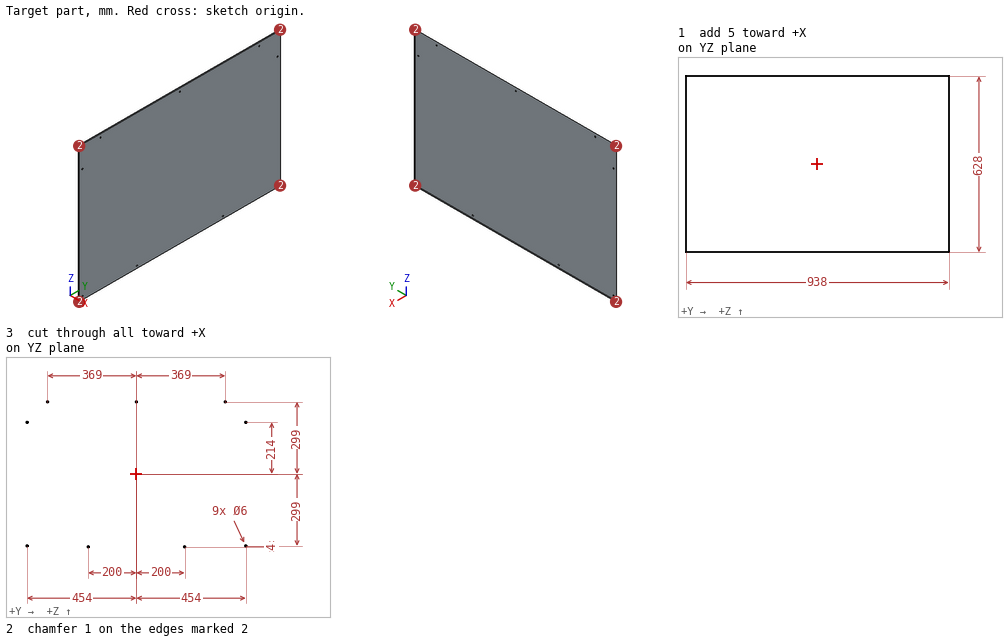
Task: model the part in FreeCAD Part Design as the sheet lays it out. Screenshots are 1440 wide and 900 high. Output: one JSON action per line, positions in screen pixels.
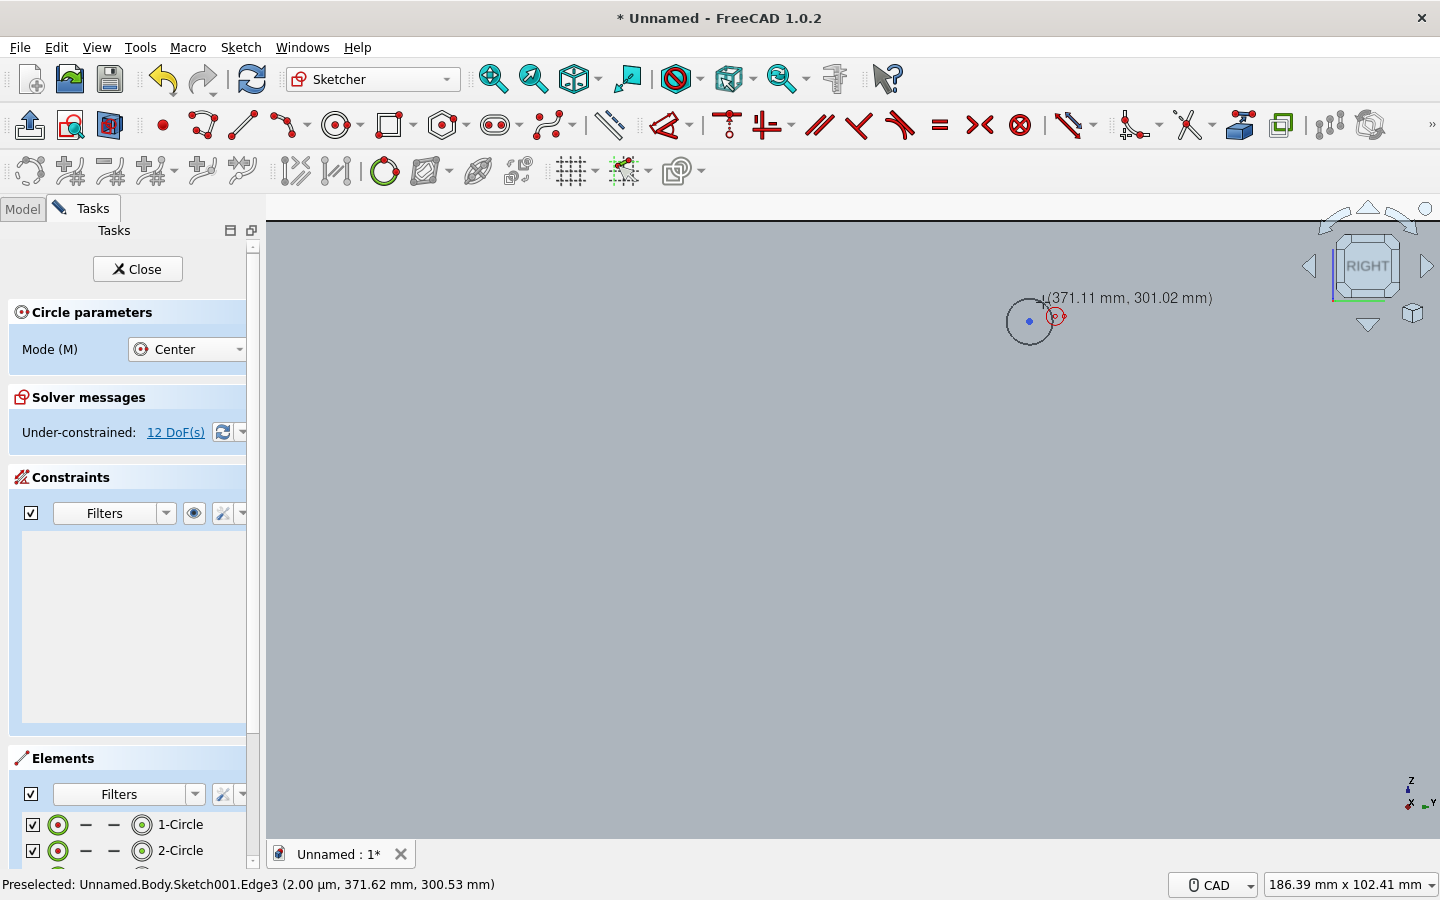
{"action": "scroll", "coordinate": [1044, 305], "scroll_direction": "down", "scroll_amount": 11}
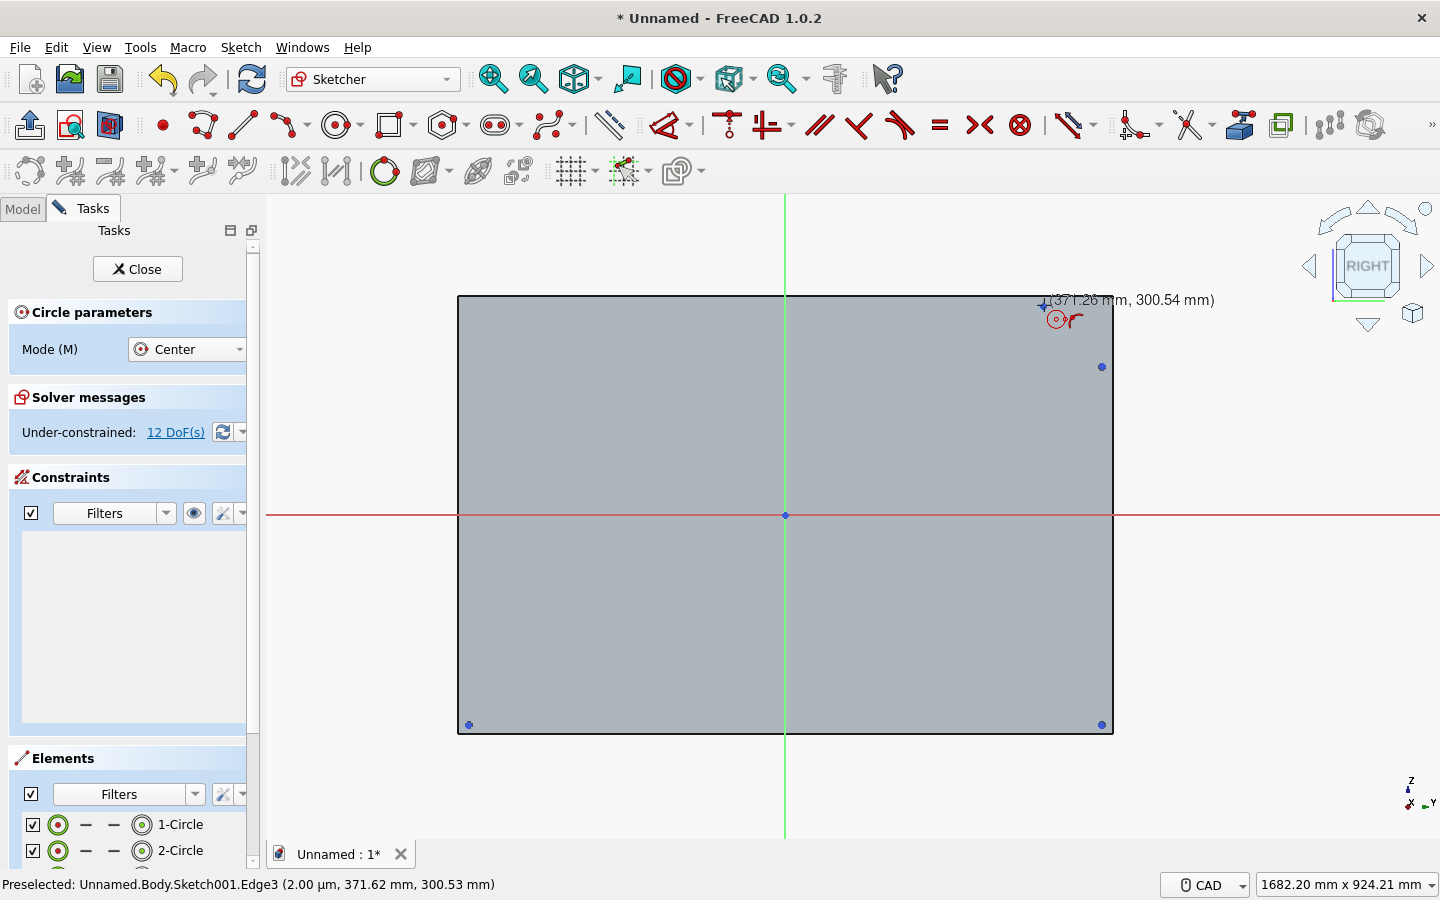
{"action": "scroll", "coordinate": [528, 306], "scroll_direction": "up", "scroll_amount": 12}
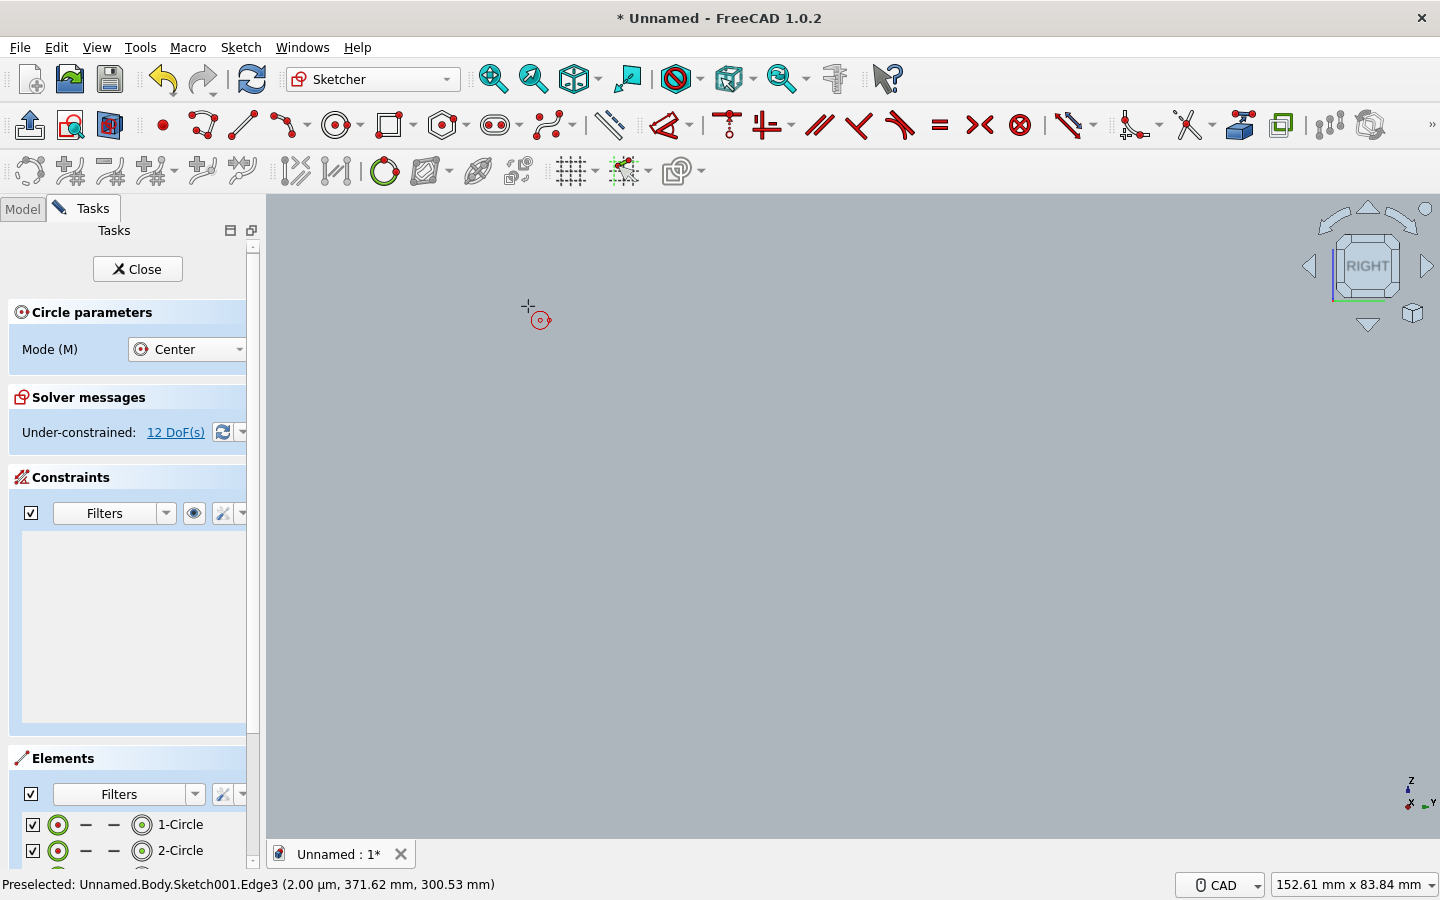
{"action": "scroll", "coordinate": [527, 306], "scroll_direction": "down", "scroll_amount": 12}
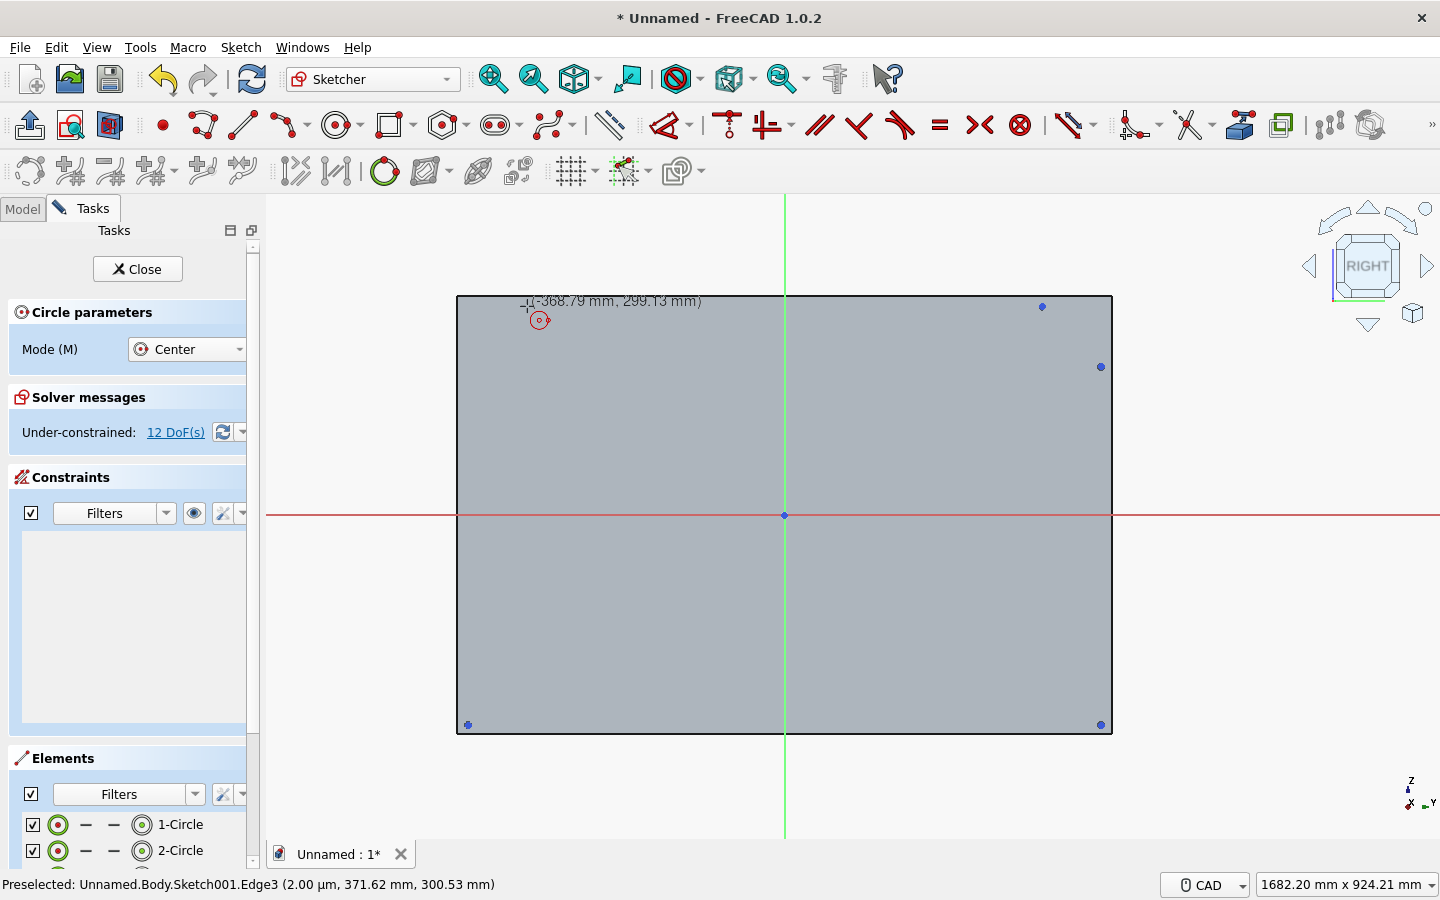
{"action": "left_click", "coordinate": [527, 306]}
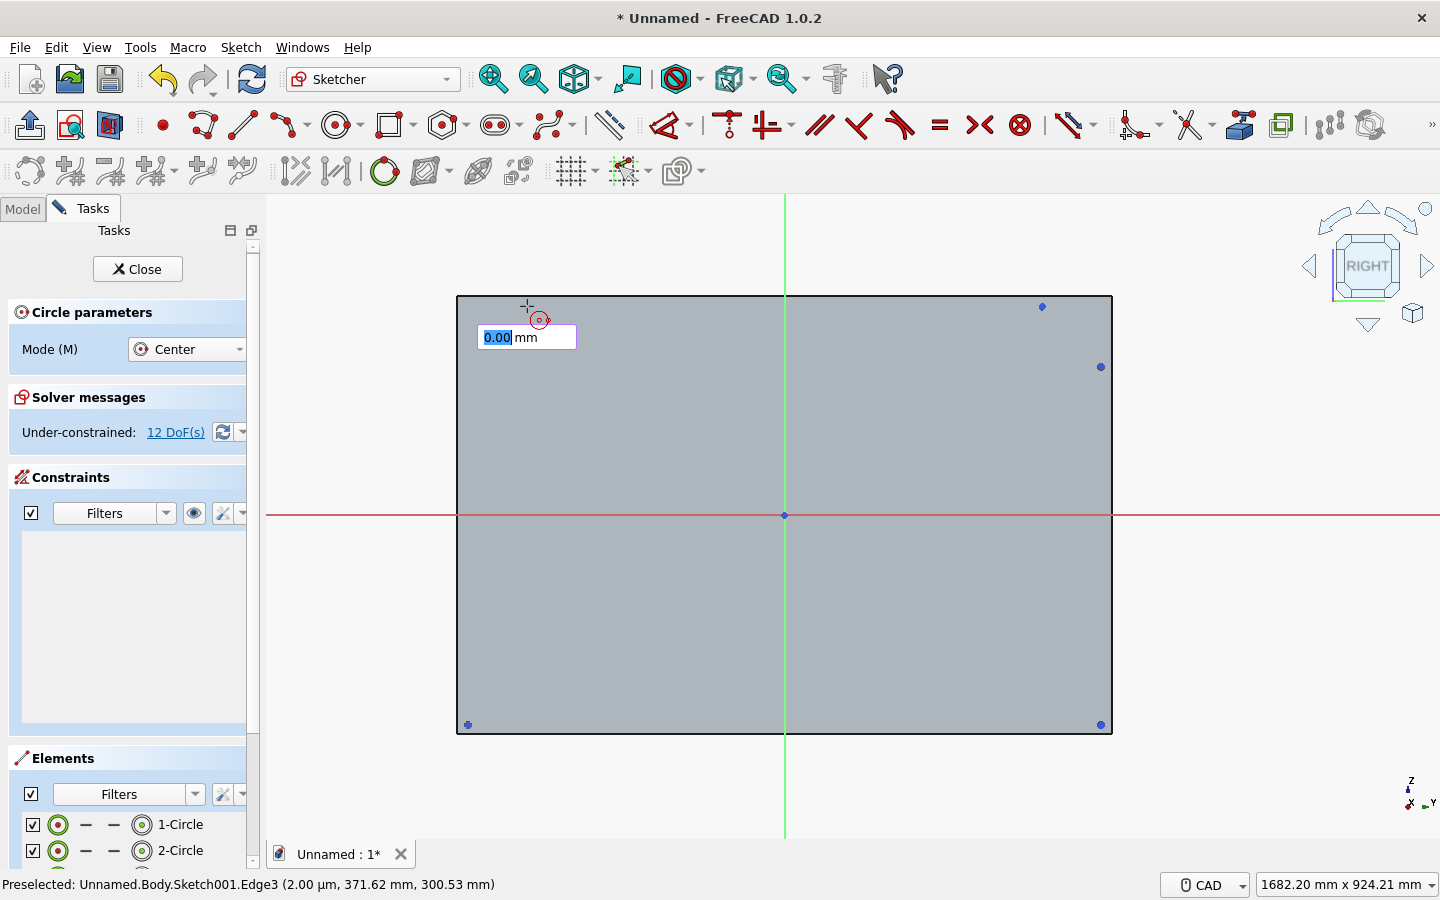
{"action": "scroll", "coordinate": [529, 305], "scroll_direction": "up", "scroll_amount": 11}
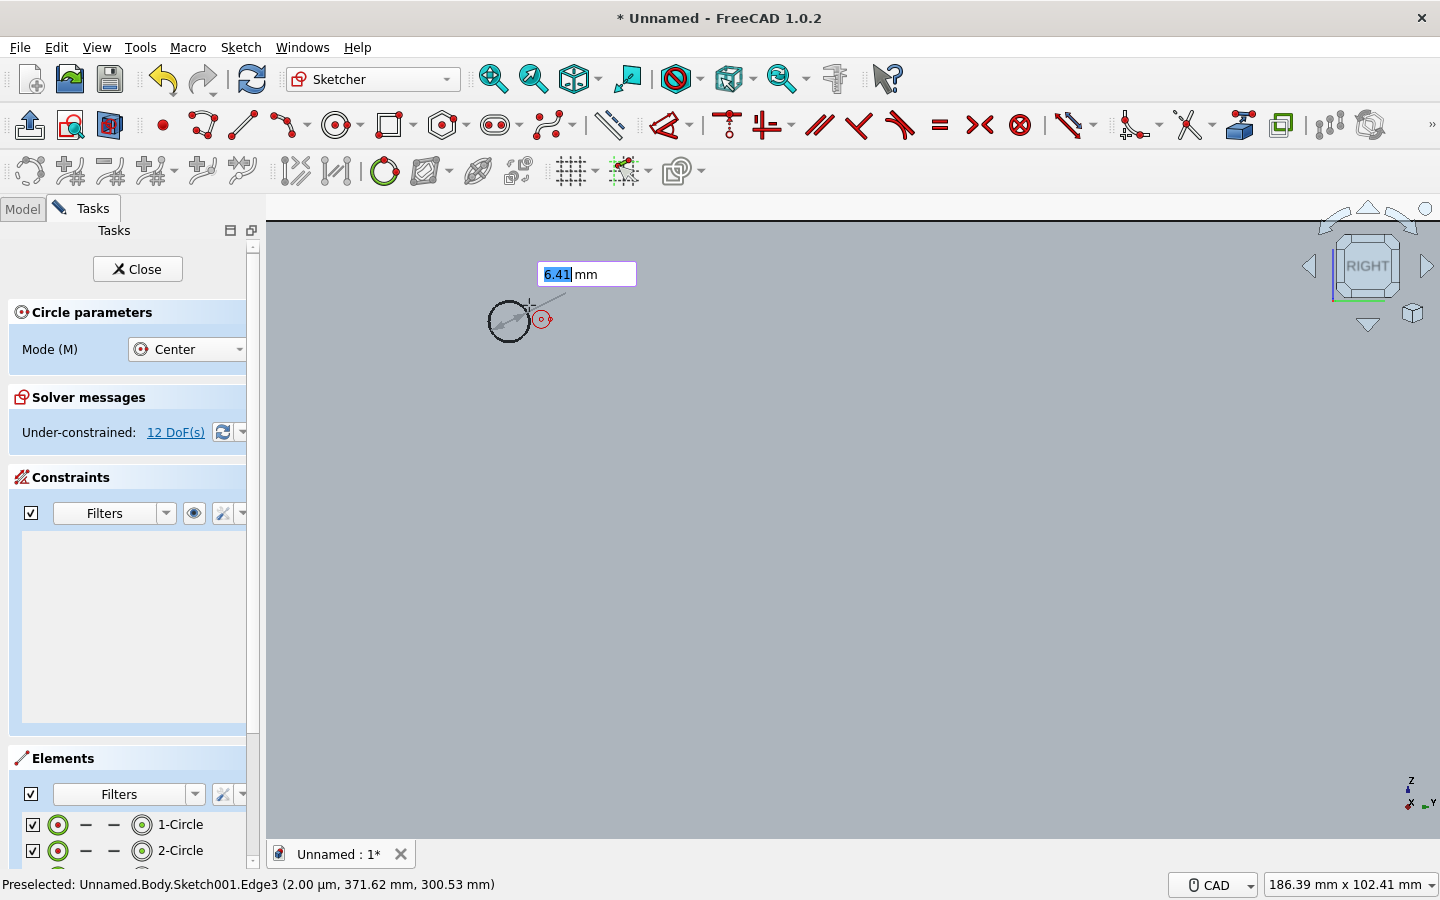
{"action": "left_click", "coordinate": [523, 302]}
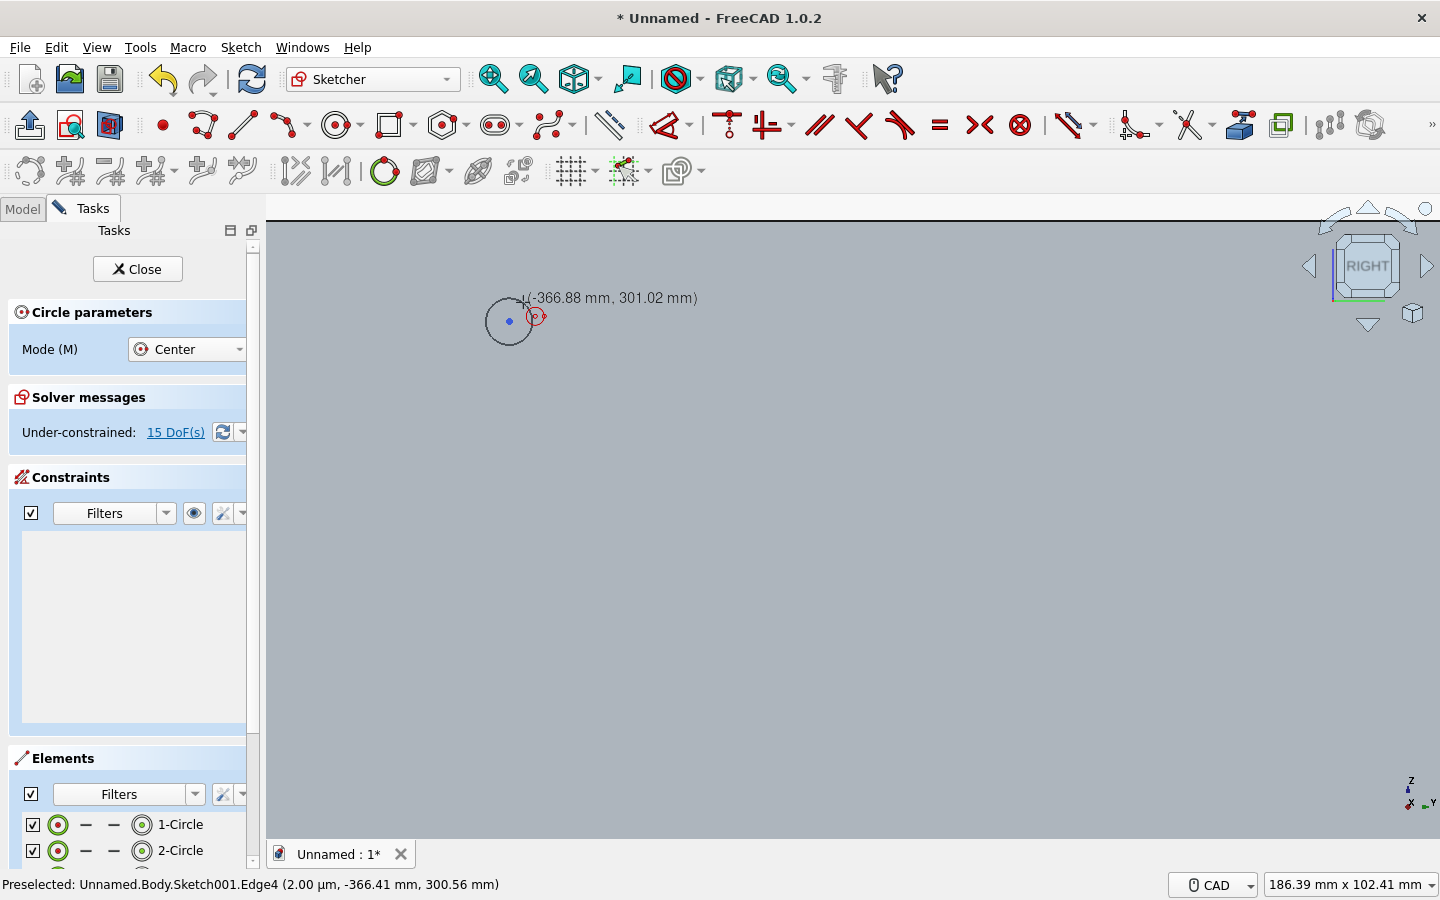
{"action": "scroll", "coordinate": [529, 305], "scroll_direction": "down", "scroll_amount": 11}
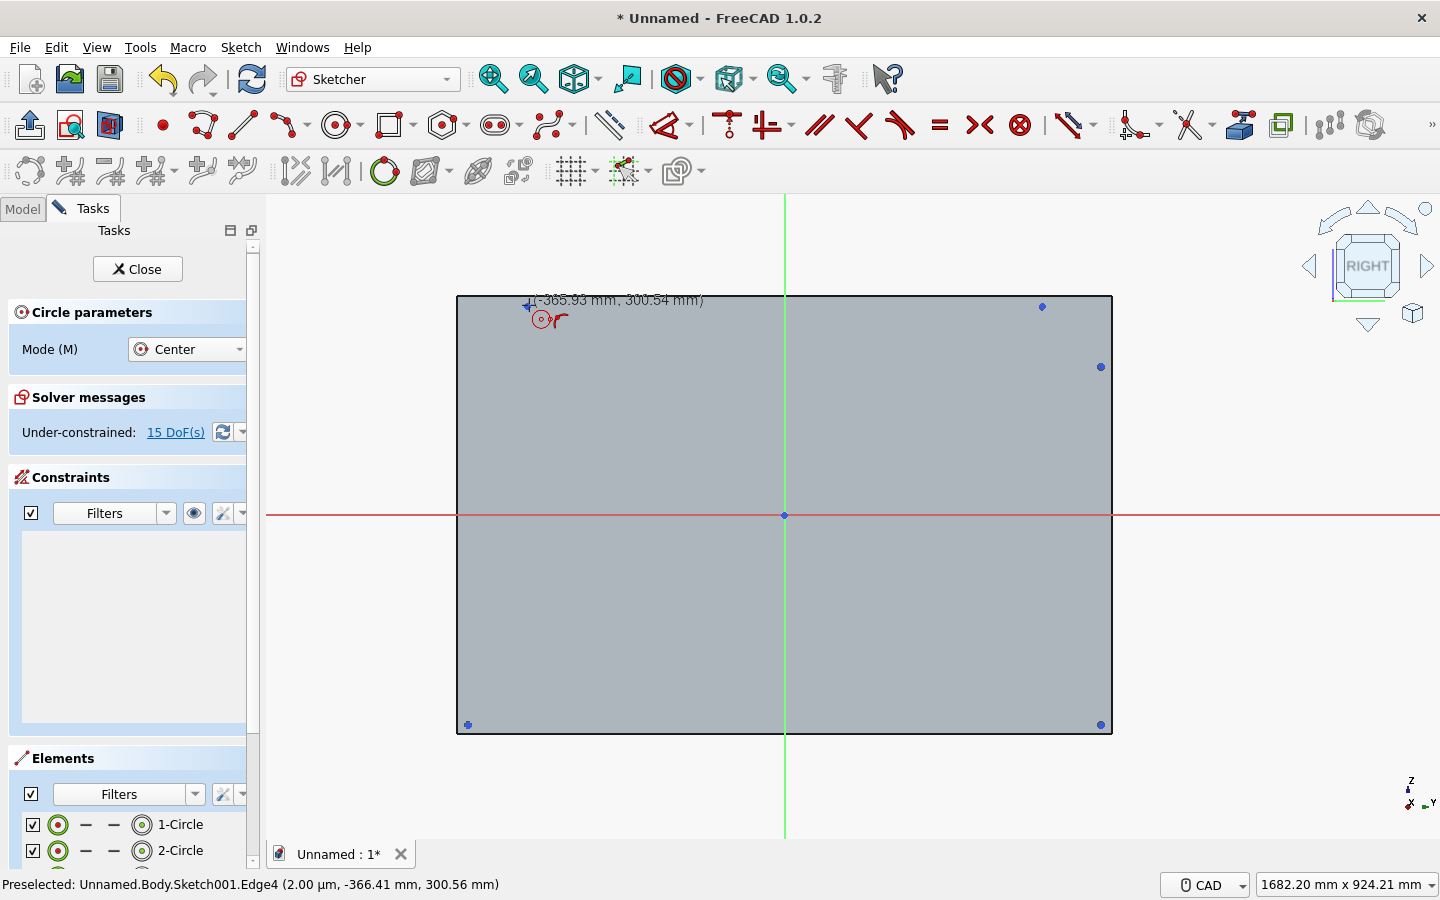
{"action": "scroll", "coordinate": [468, 366], "scroll_direction": "up", "scroll_amount": 12}